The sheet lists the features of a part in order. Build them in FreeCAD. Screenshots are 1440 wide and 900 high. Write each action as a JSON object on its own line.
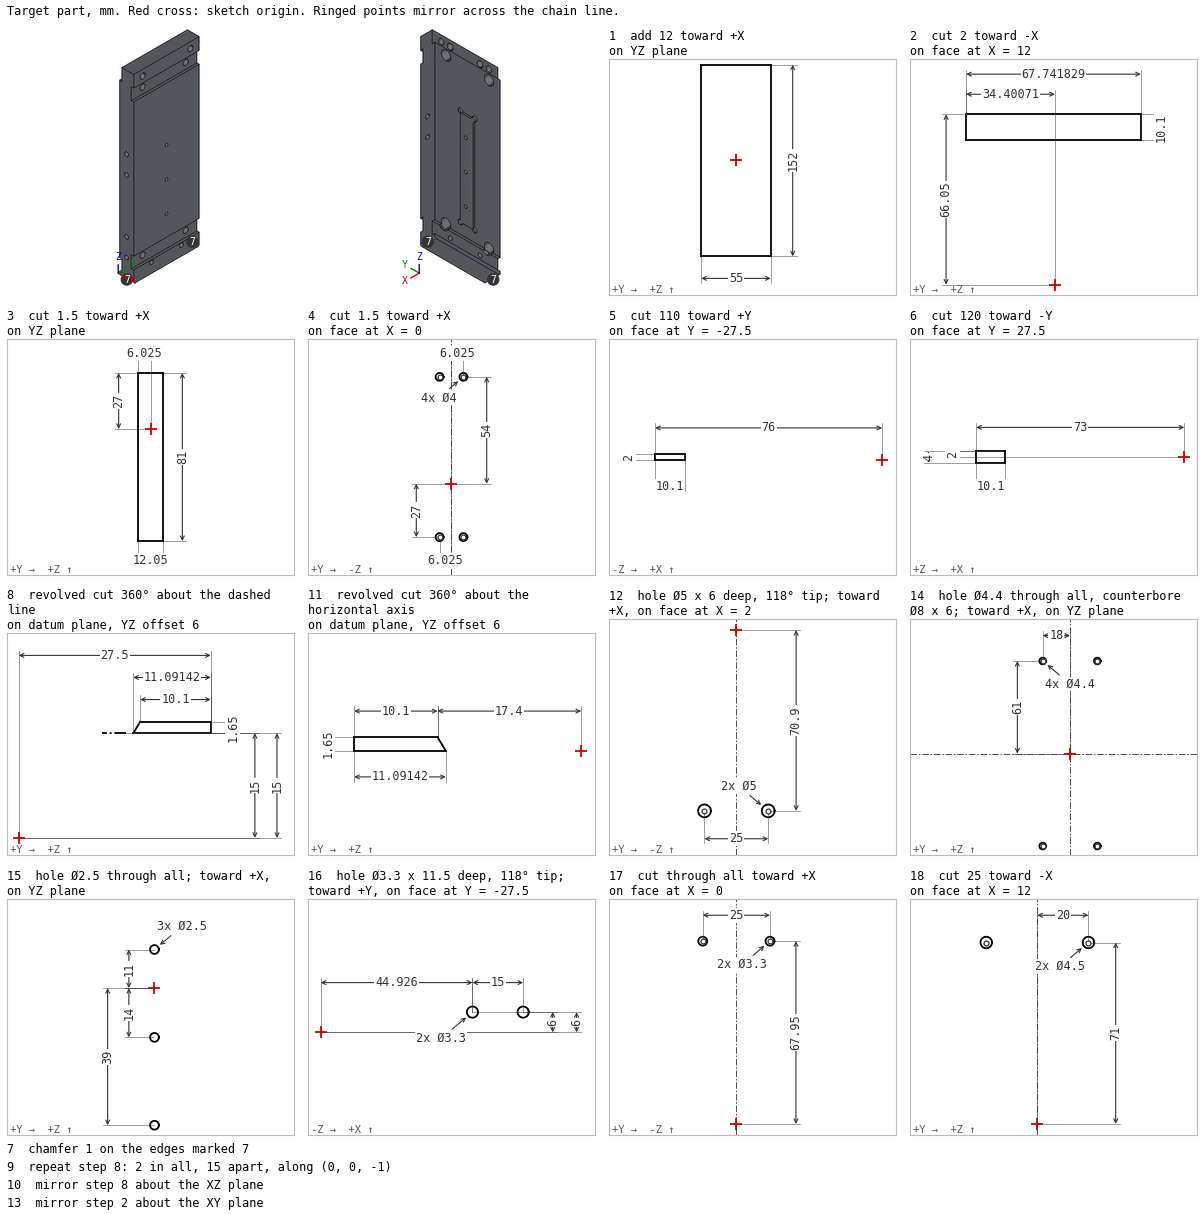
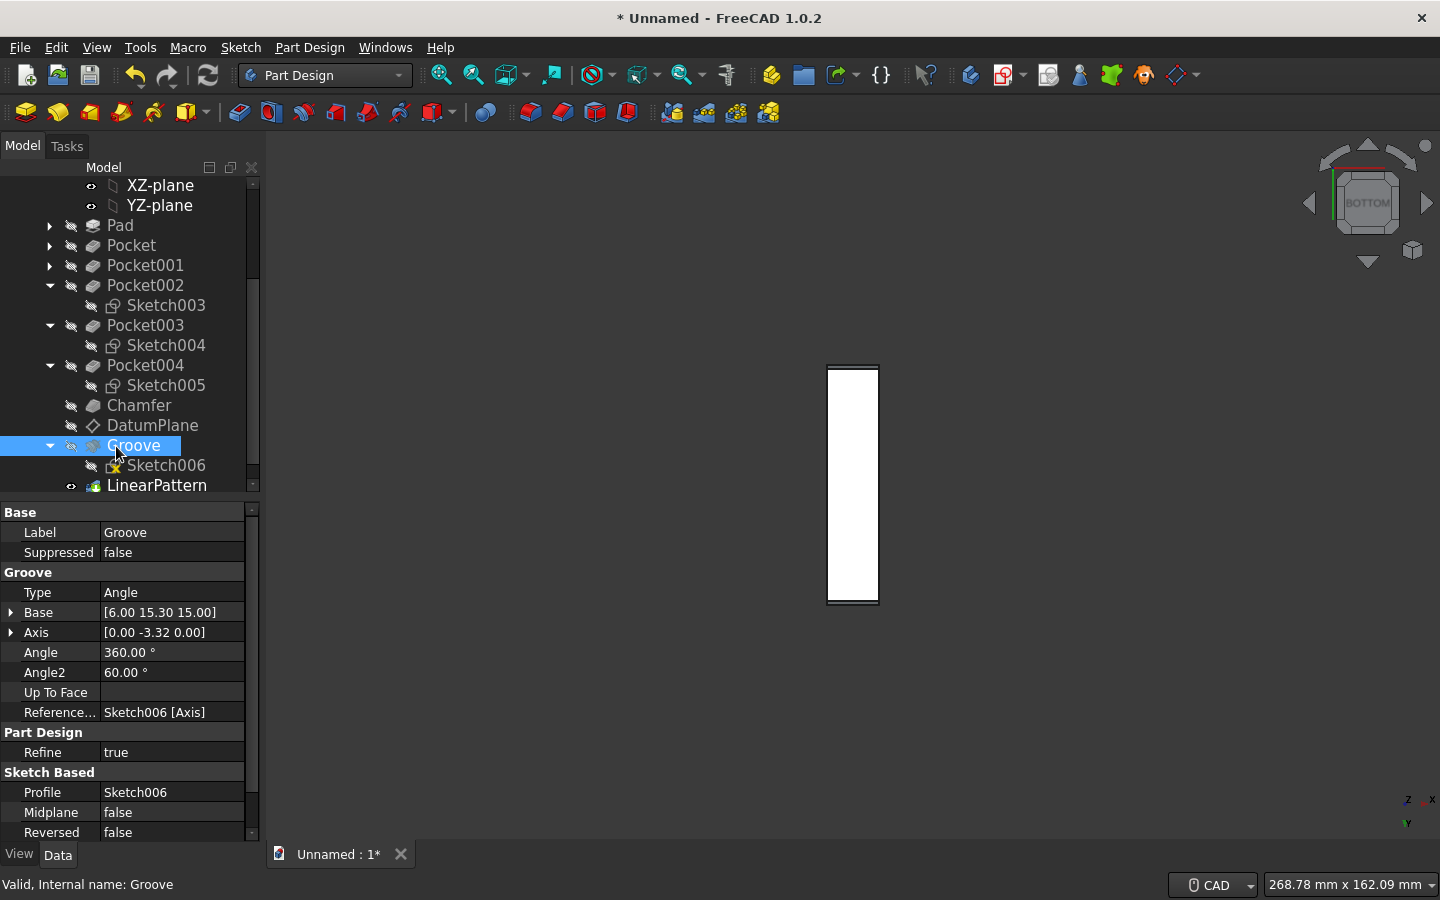
{"action": "left_click", "coordinate": [672, 112]}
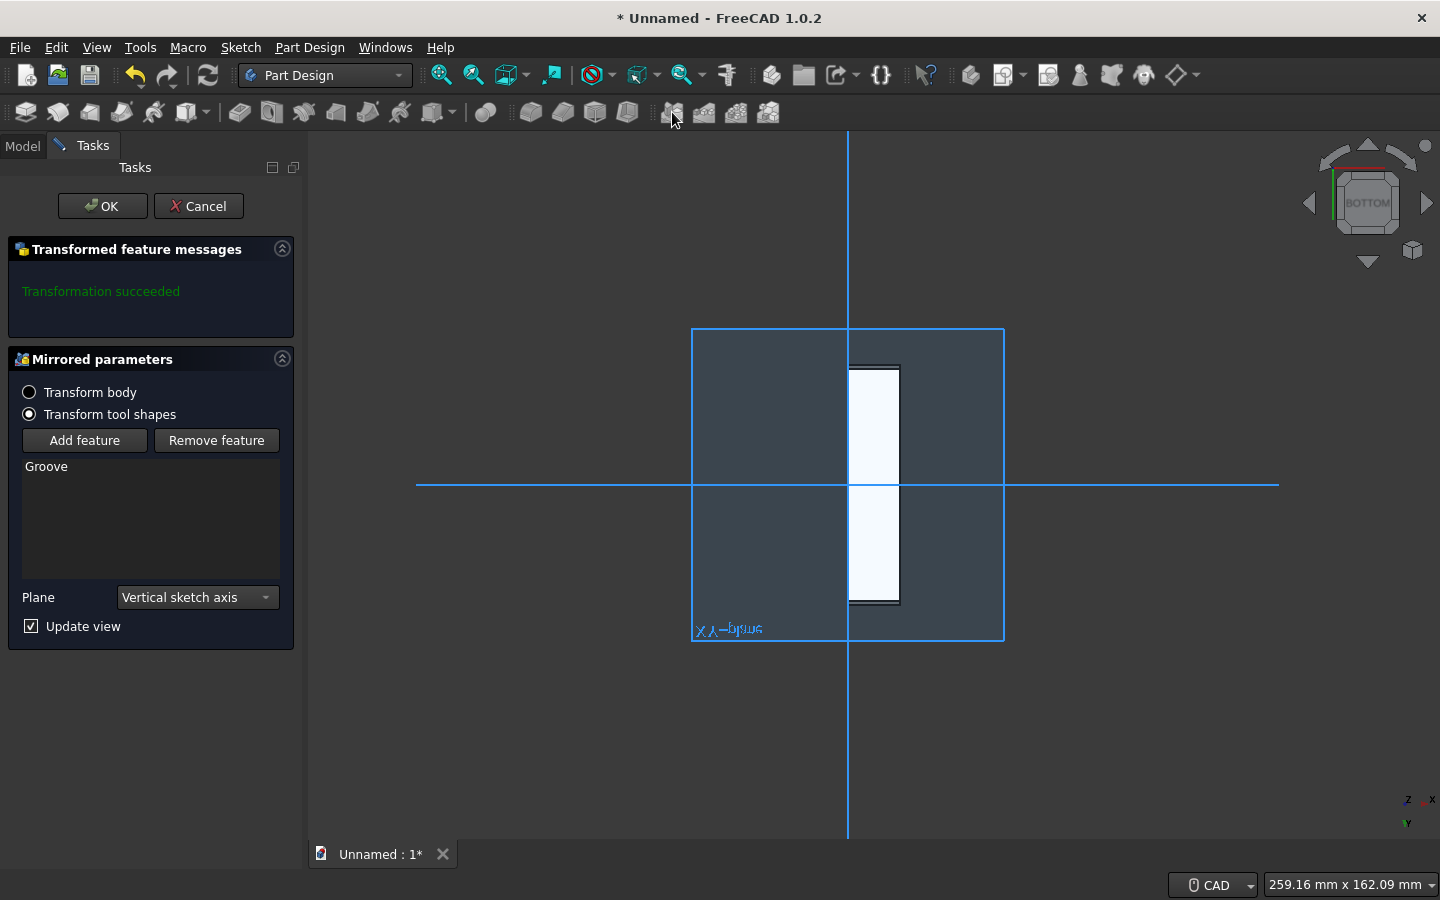
{"action": "left_click", "coordinate": [198, 598]}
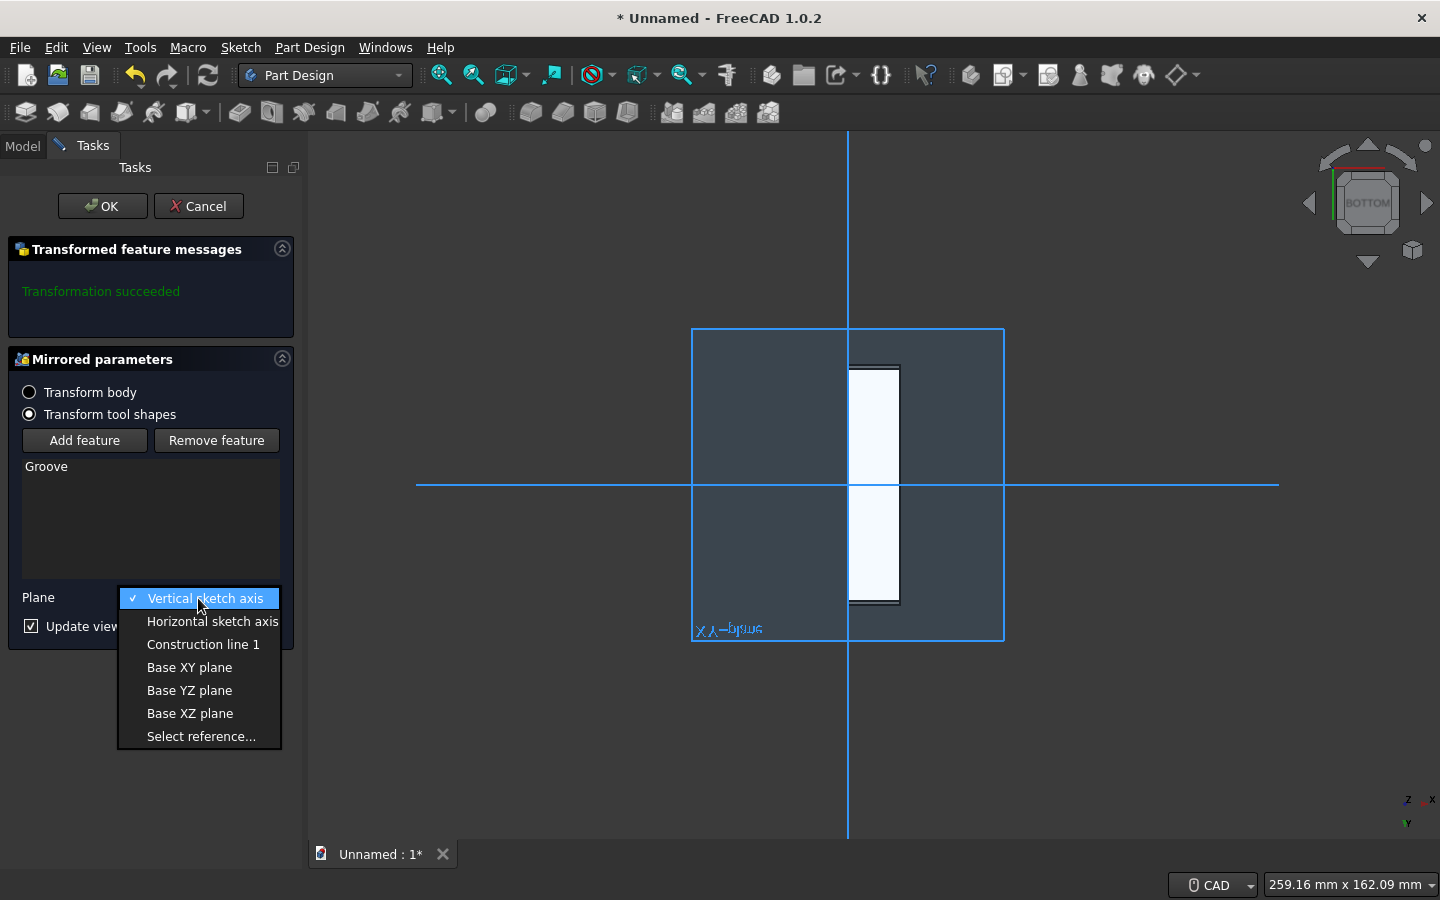
{"action": "left_click", "coordinate": [198, 714]}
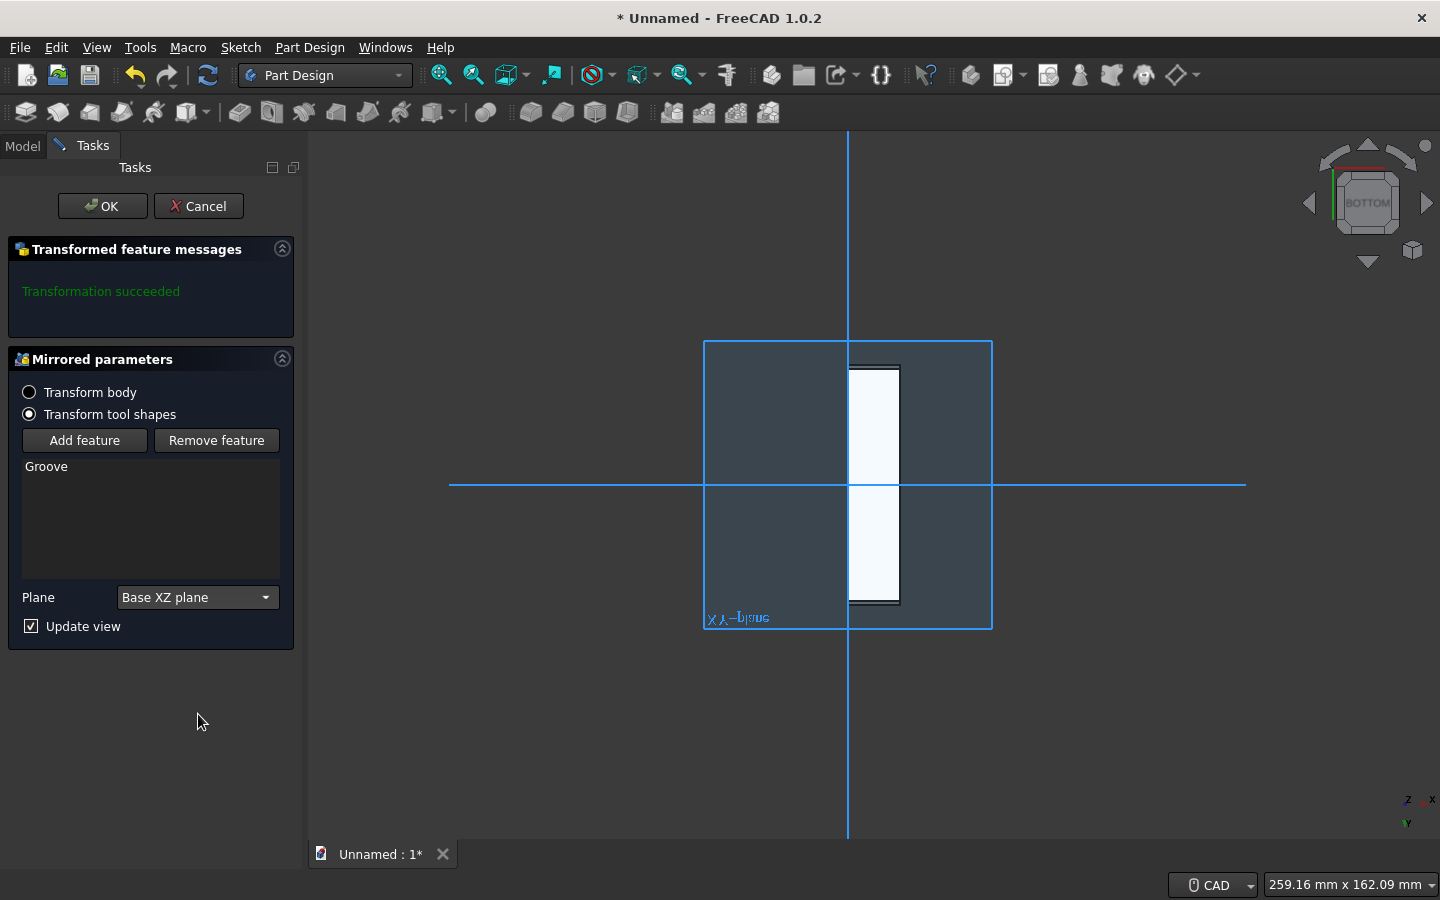
{"action": "left_click", "coordinate": [103, 206]}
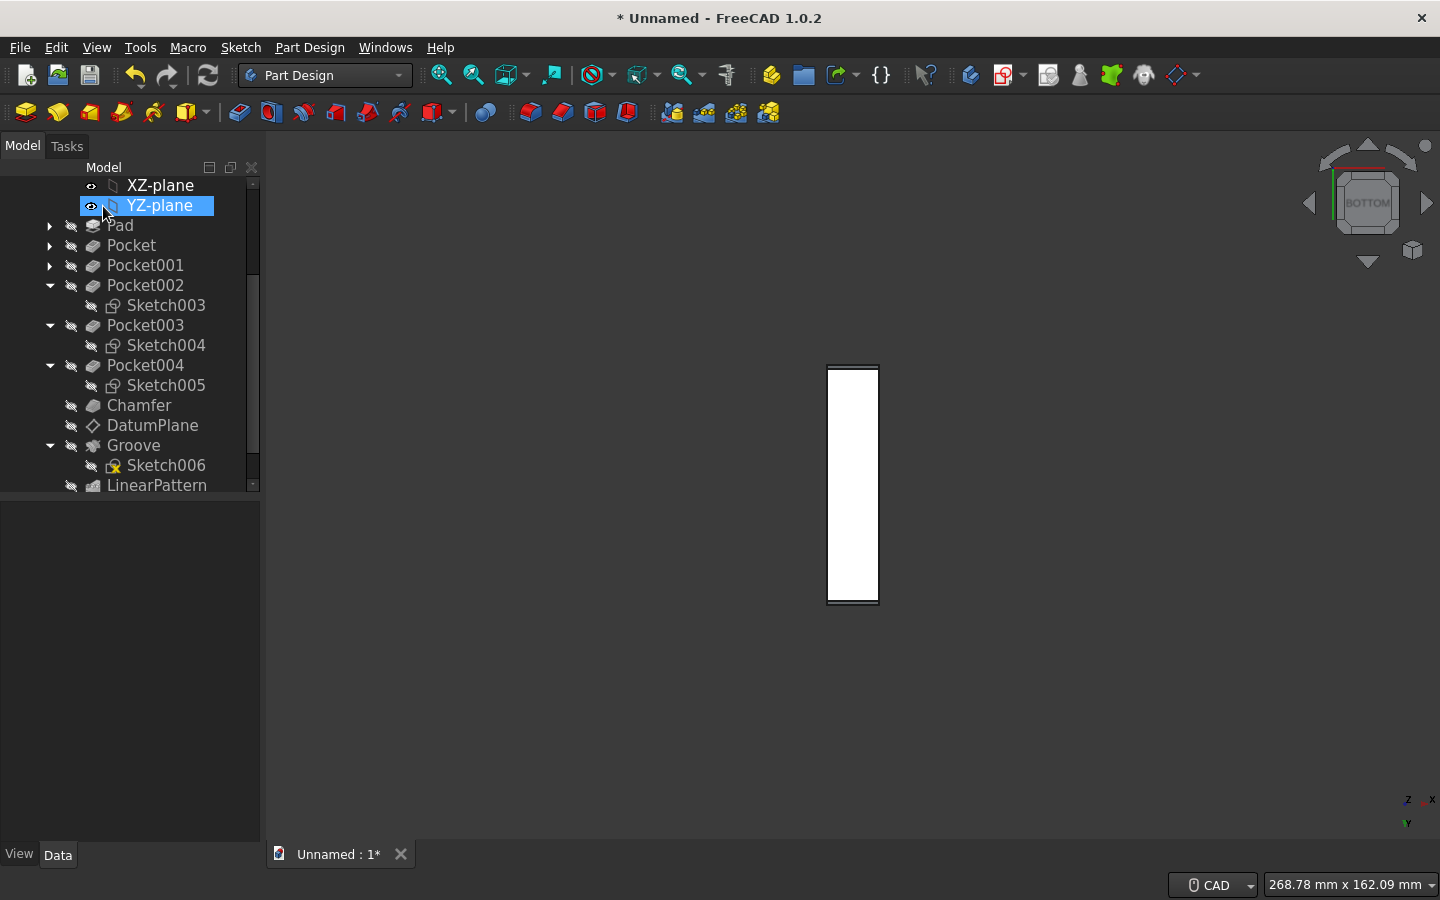
{"action": "left_click", "coordinate": [442, 76]}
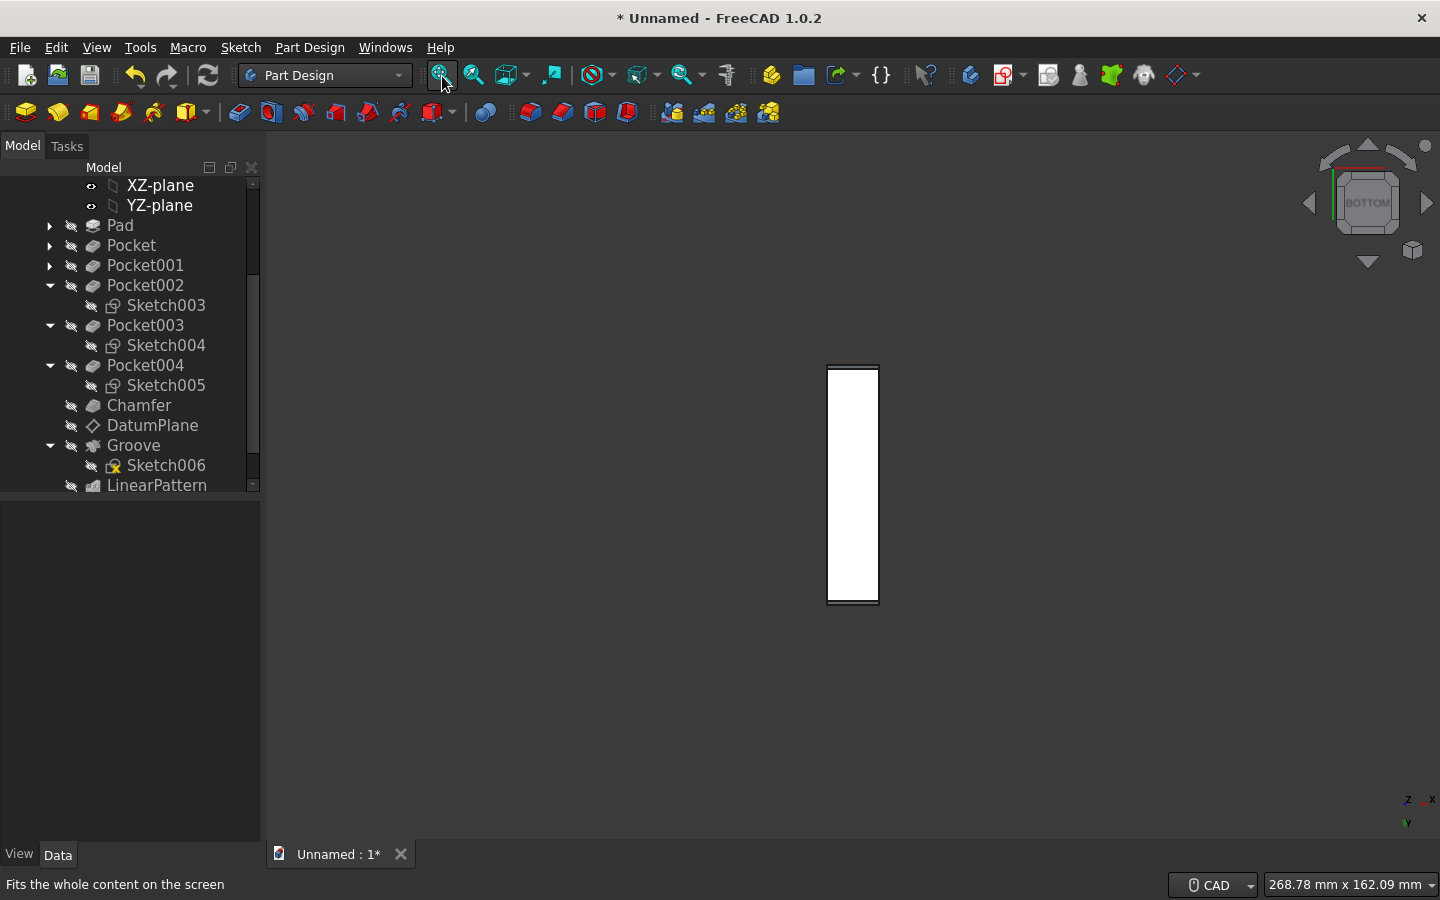
{"action": "scroll", "coordinate": [160, 341], "scroll_direction": "down", "scroll_amount": 3}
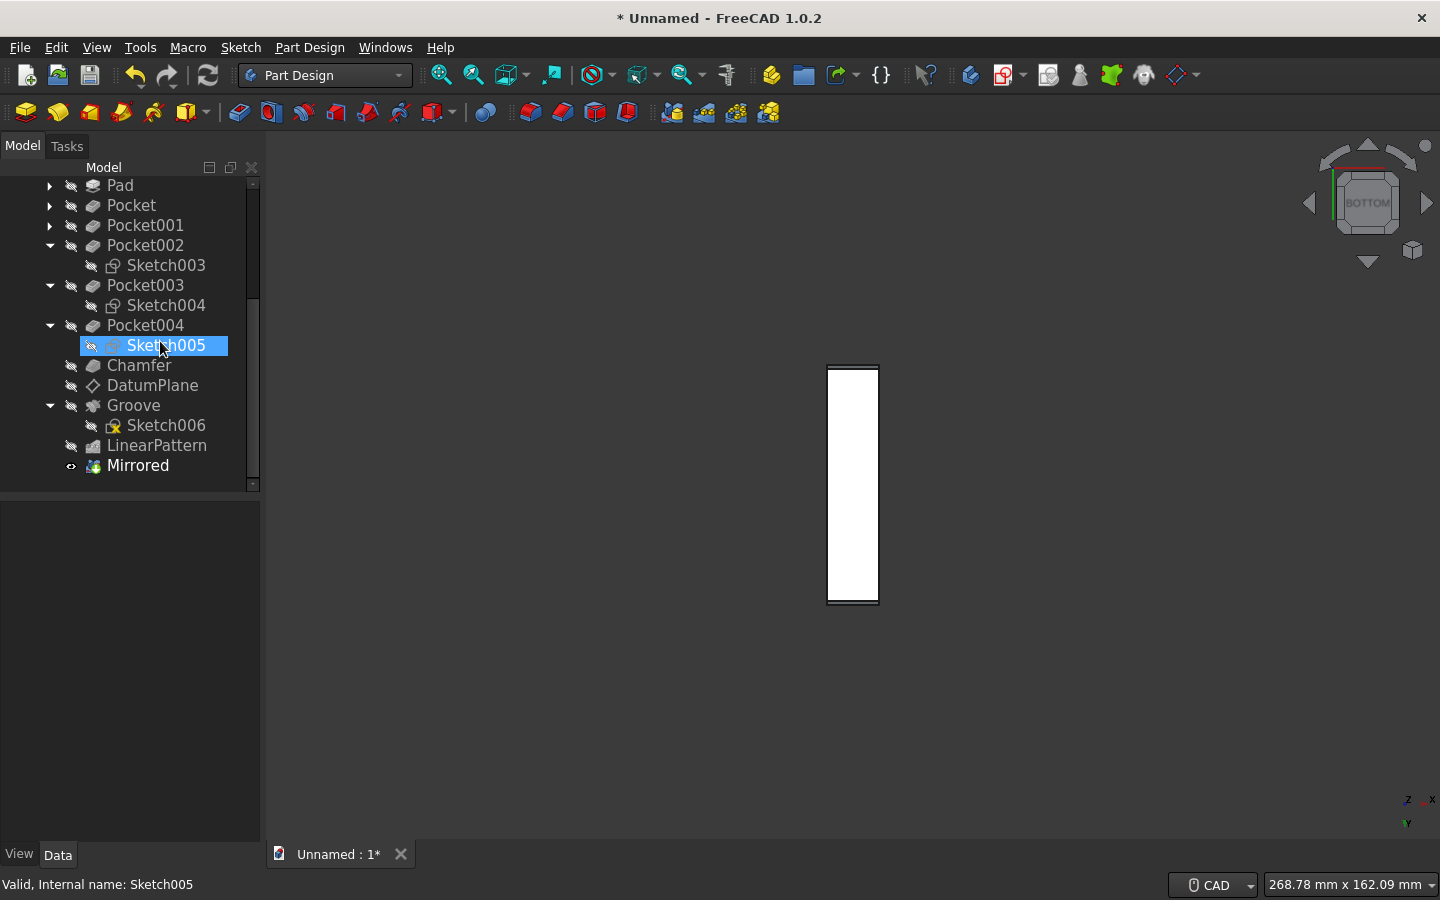
{"action": "scroll", "coordinate": [140, 321], "scroll_direction": "up", "scroll_amount": 15}